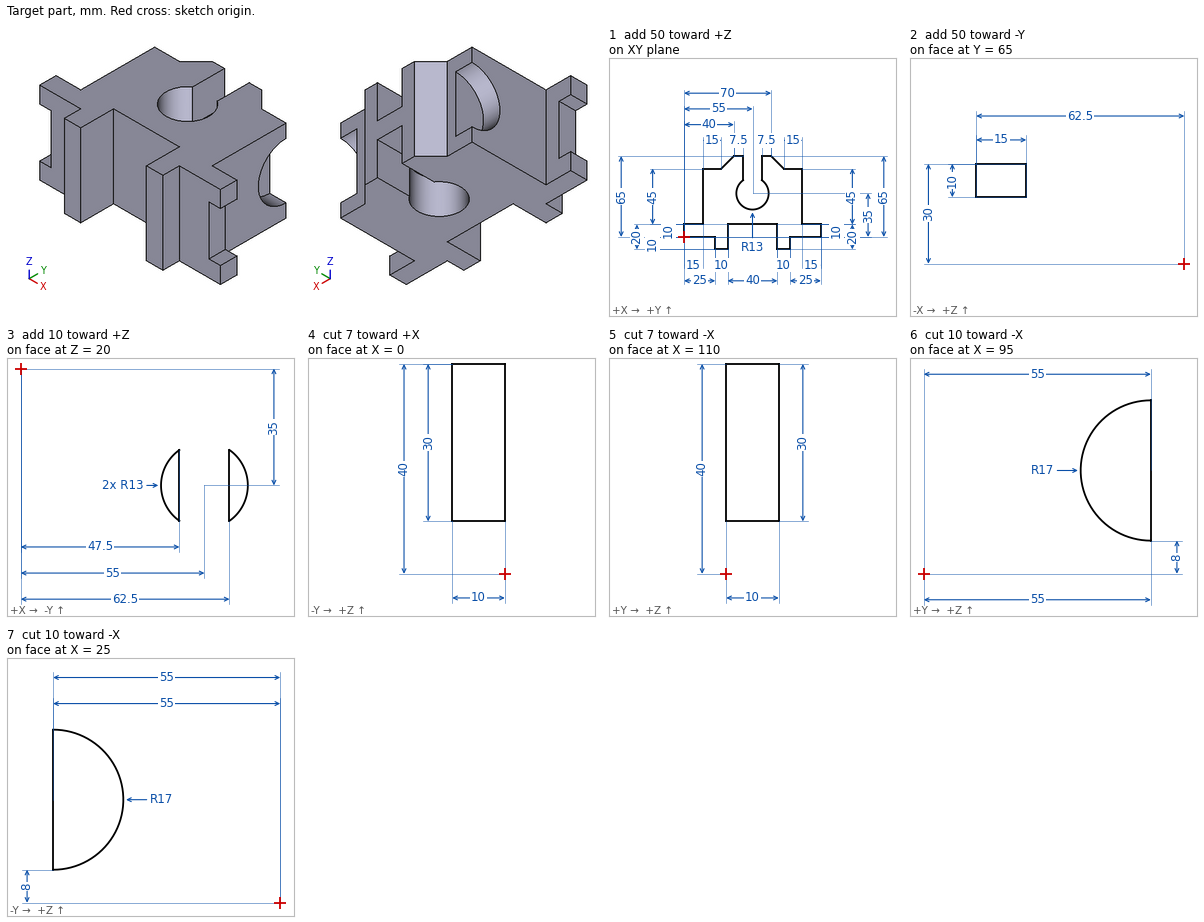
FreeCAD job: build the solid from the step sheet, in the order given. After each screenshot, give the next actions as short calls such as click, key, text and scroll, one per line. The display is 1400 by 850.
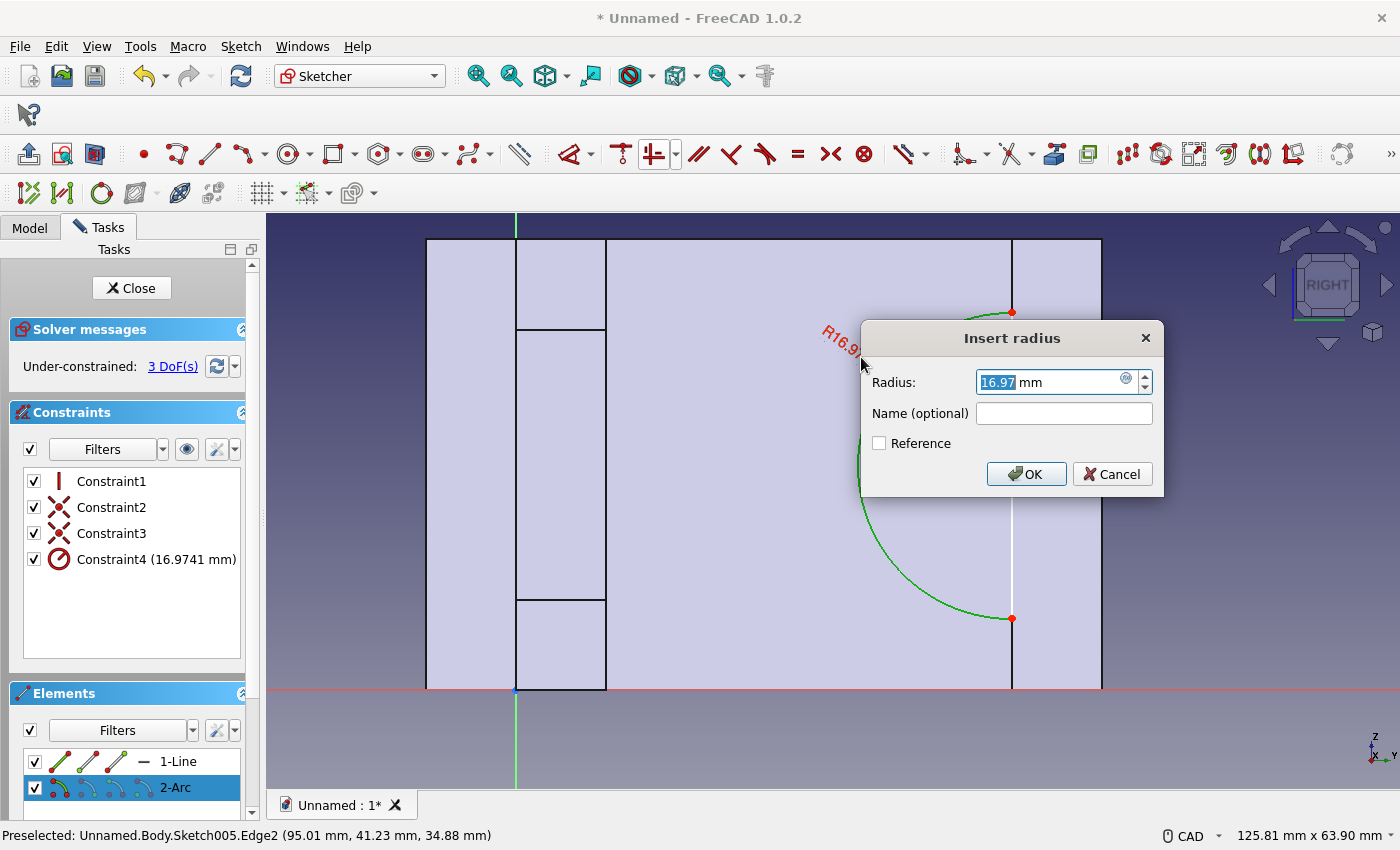
text(17)
key(Return)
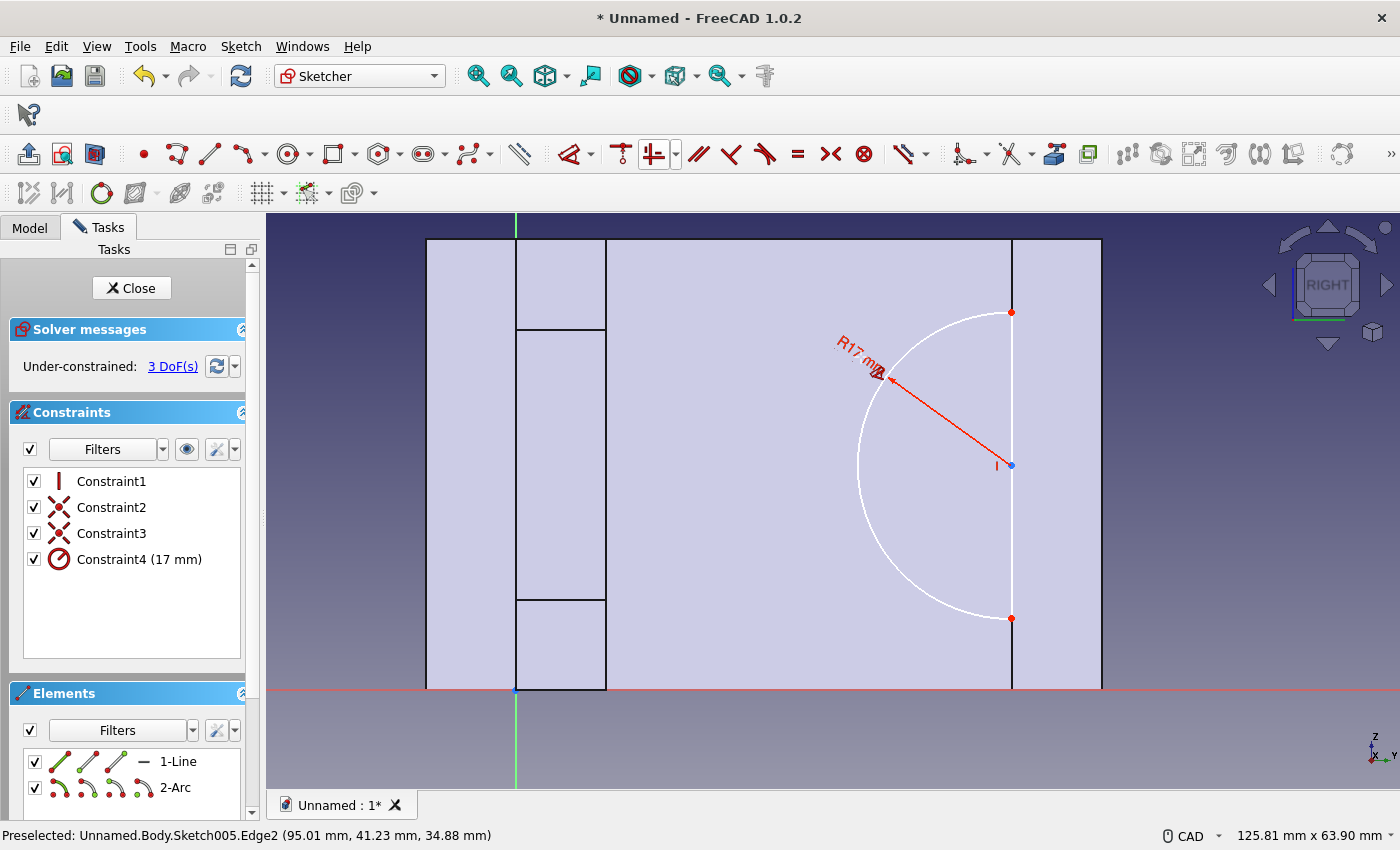
click(1012, 619)
click(1046, 655)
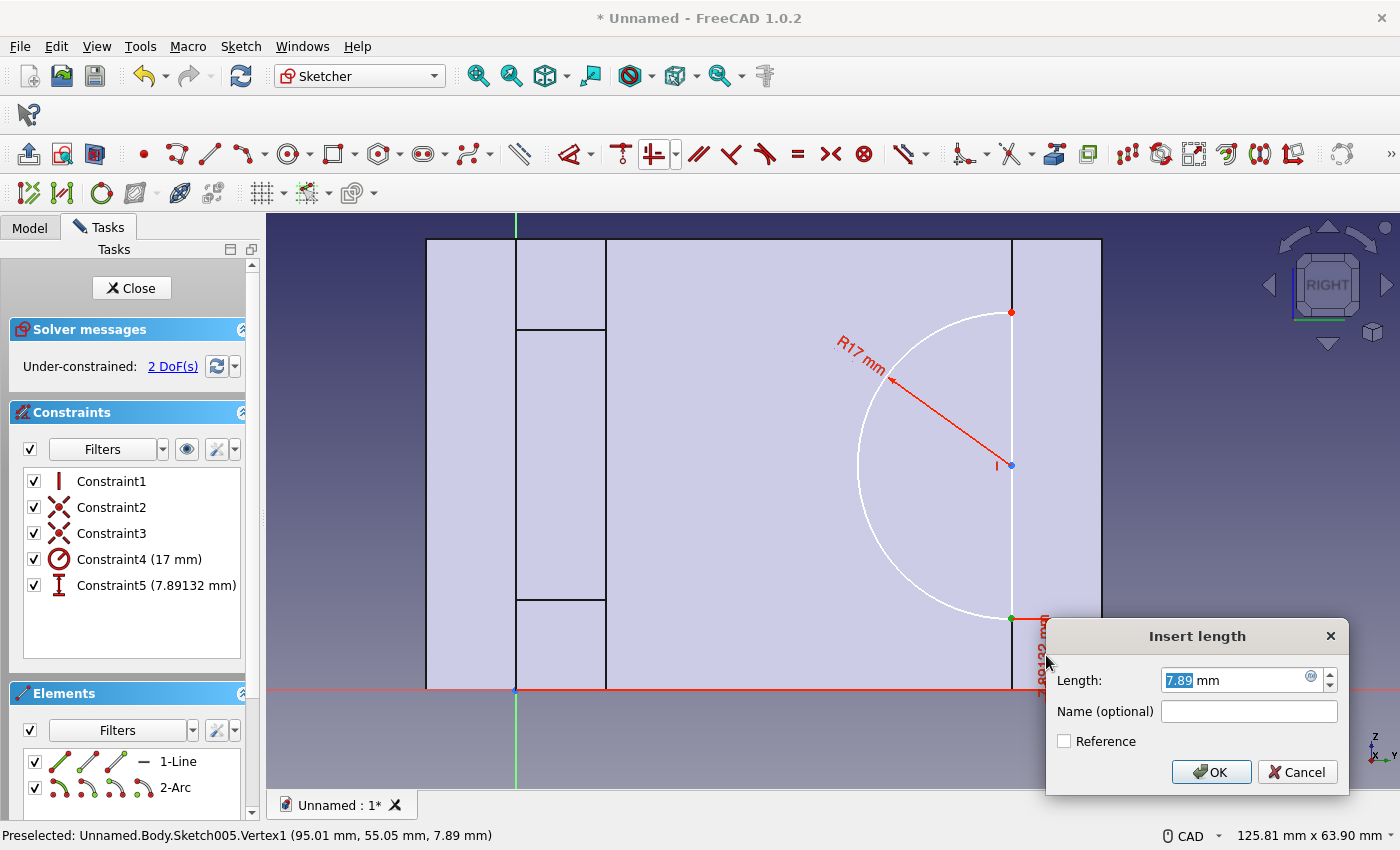
text(8)
key(Return)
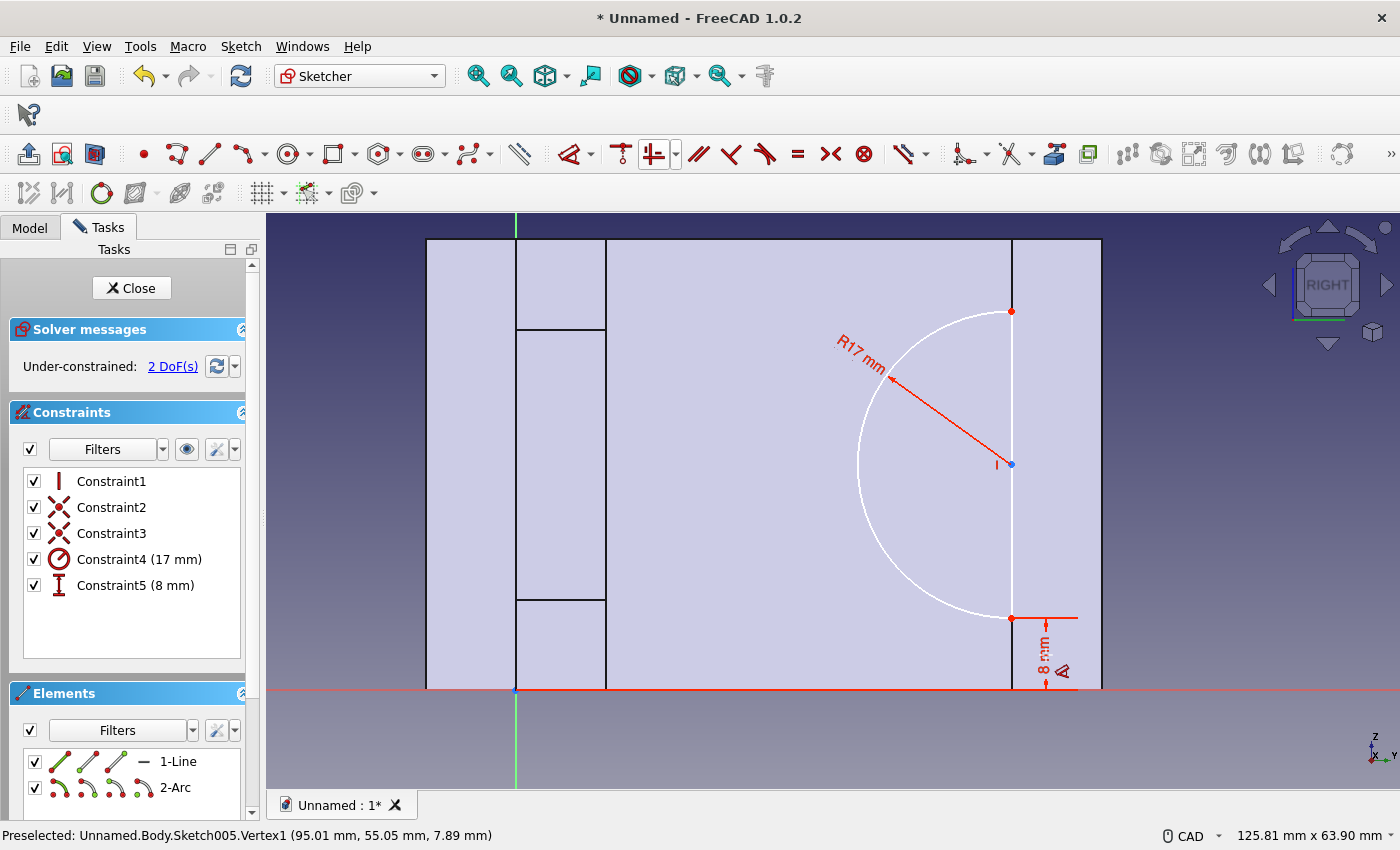
click(1012, 618)
click(764, 724)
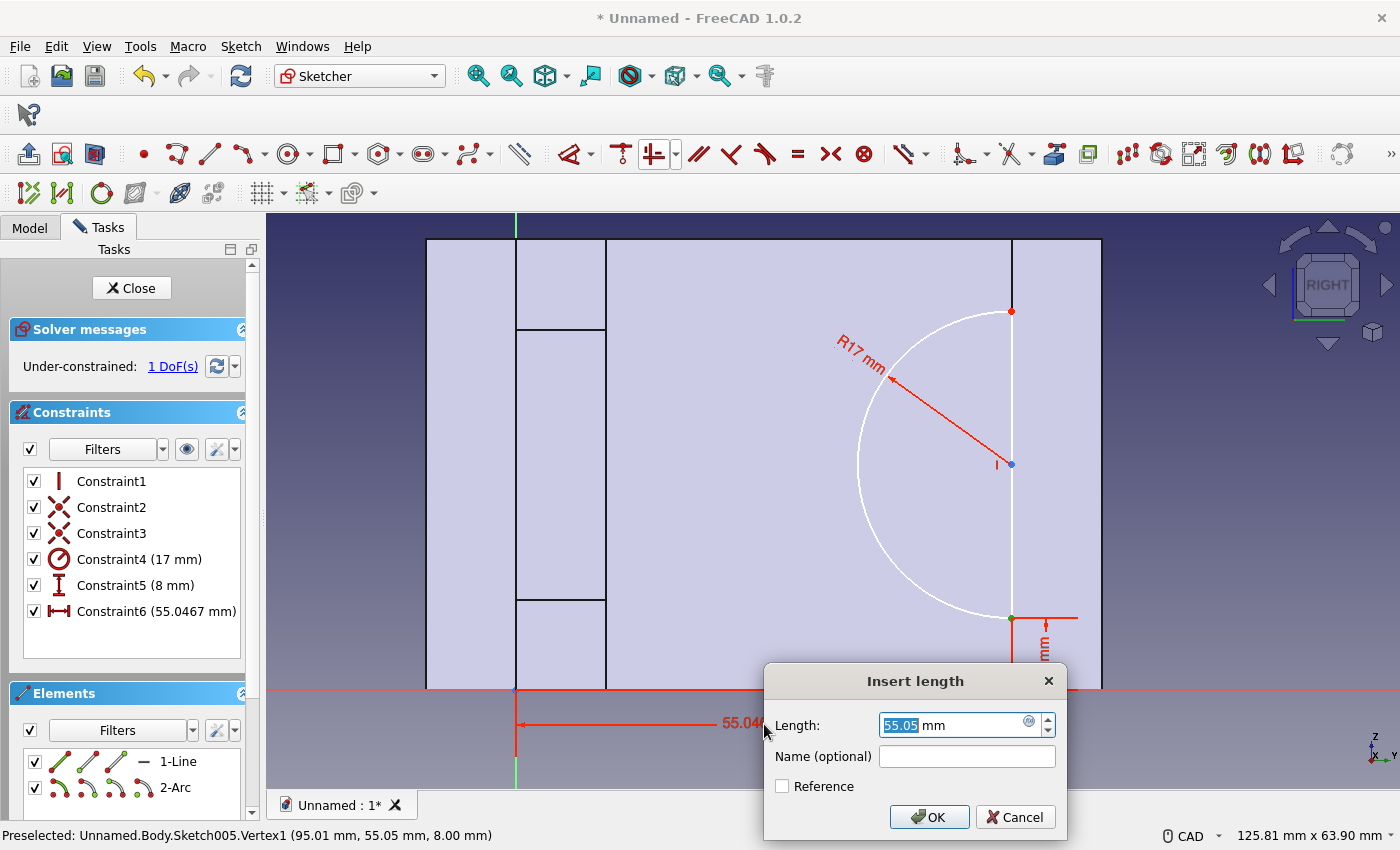
text(55)
key(Return)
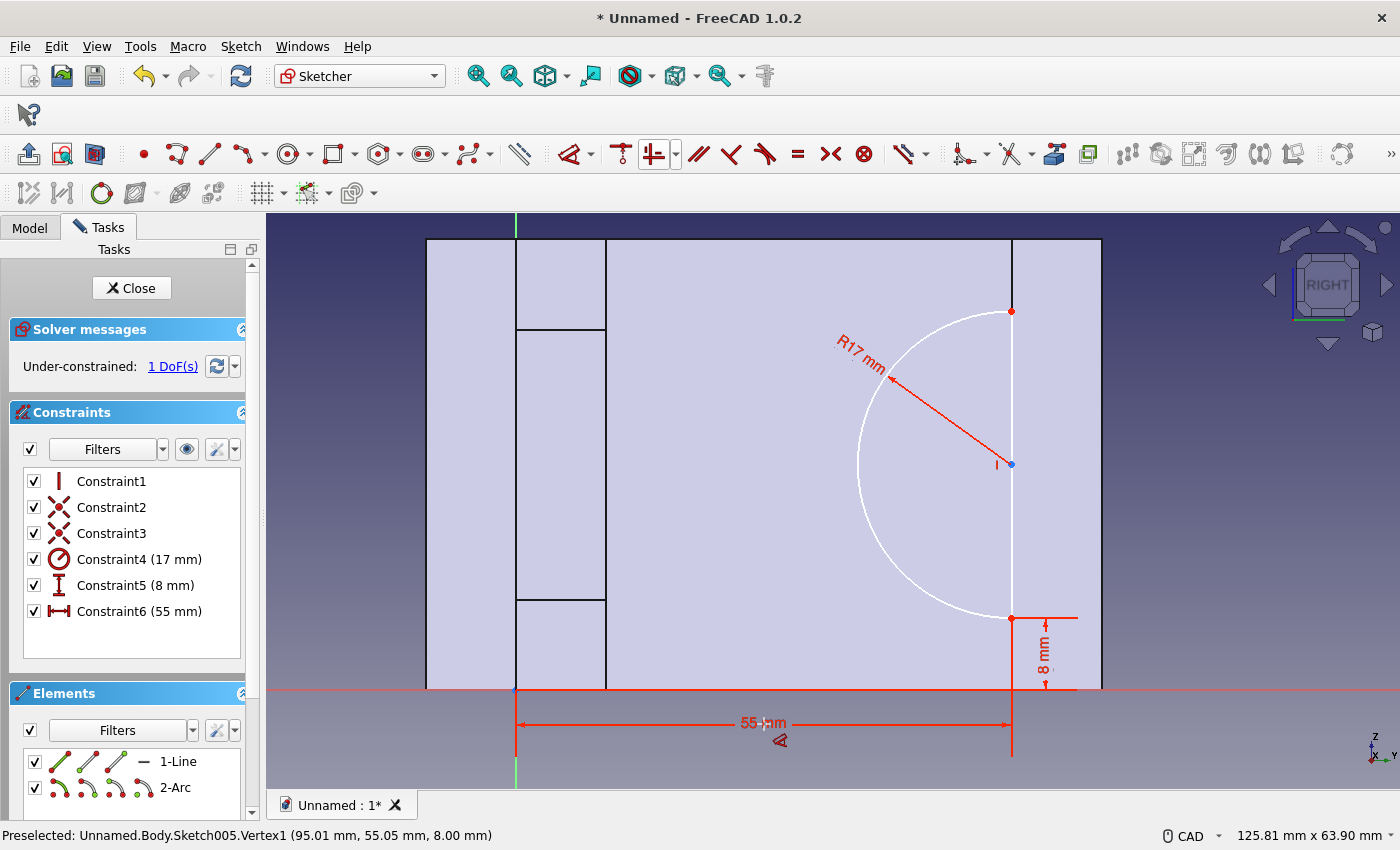
click(1011, 465)
click(650, 724)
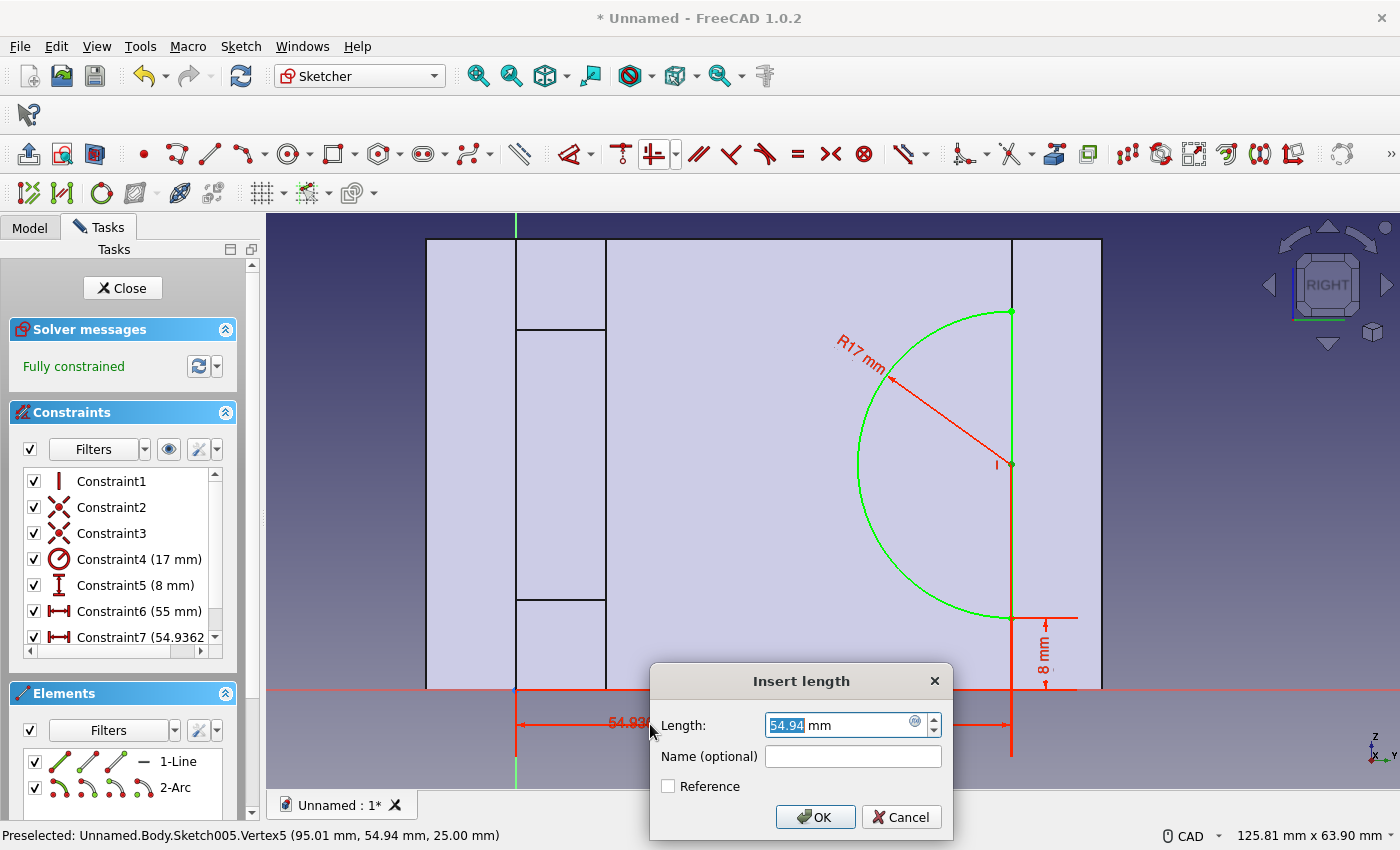
text(55)
key(Return)
key(Escape)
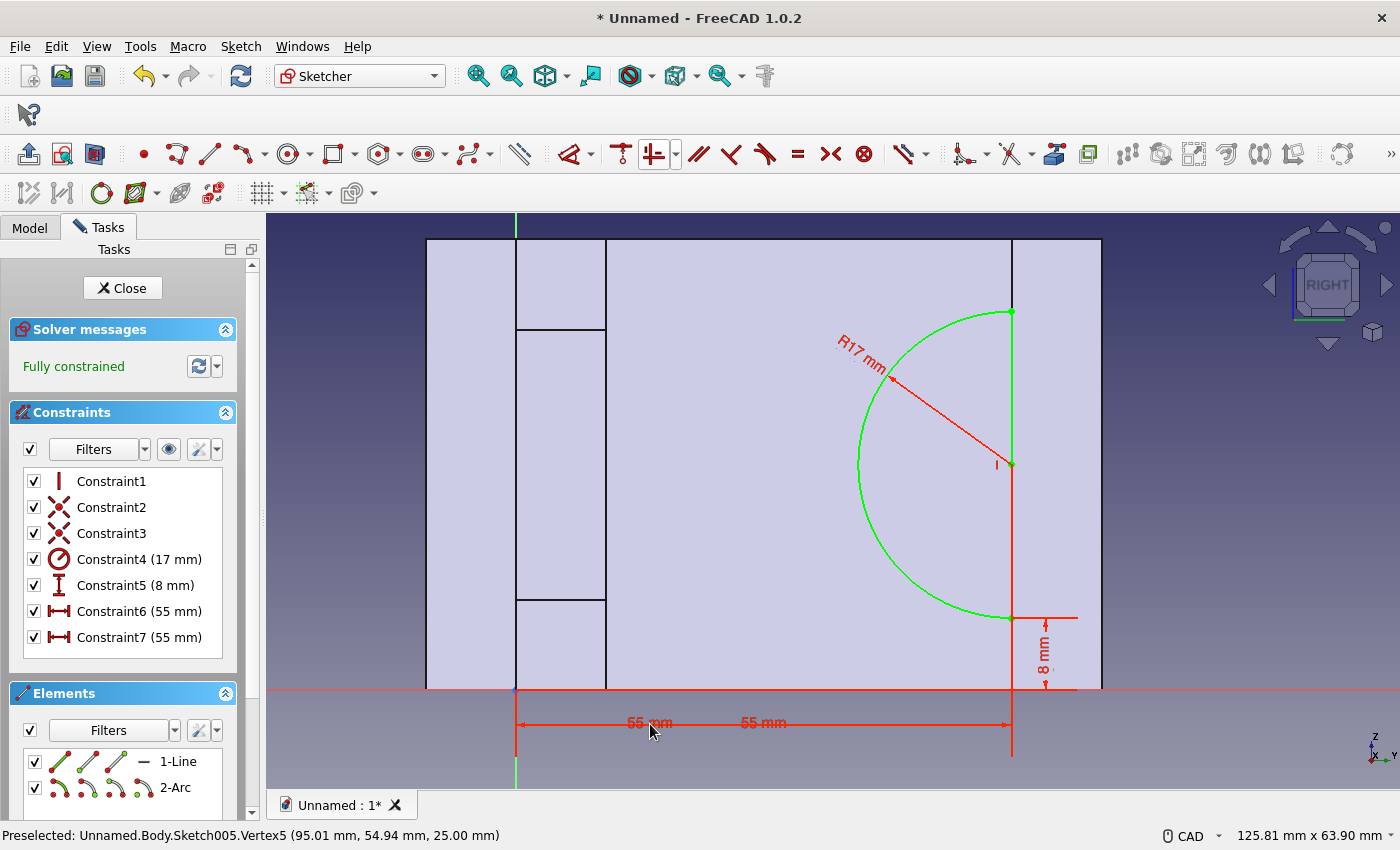
click(123, 288)